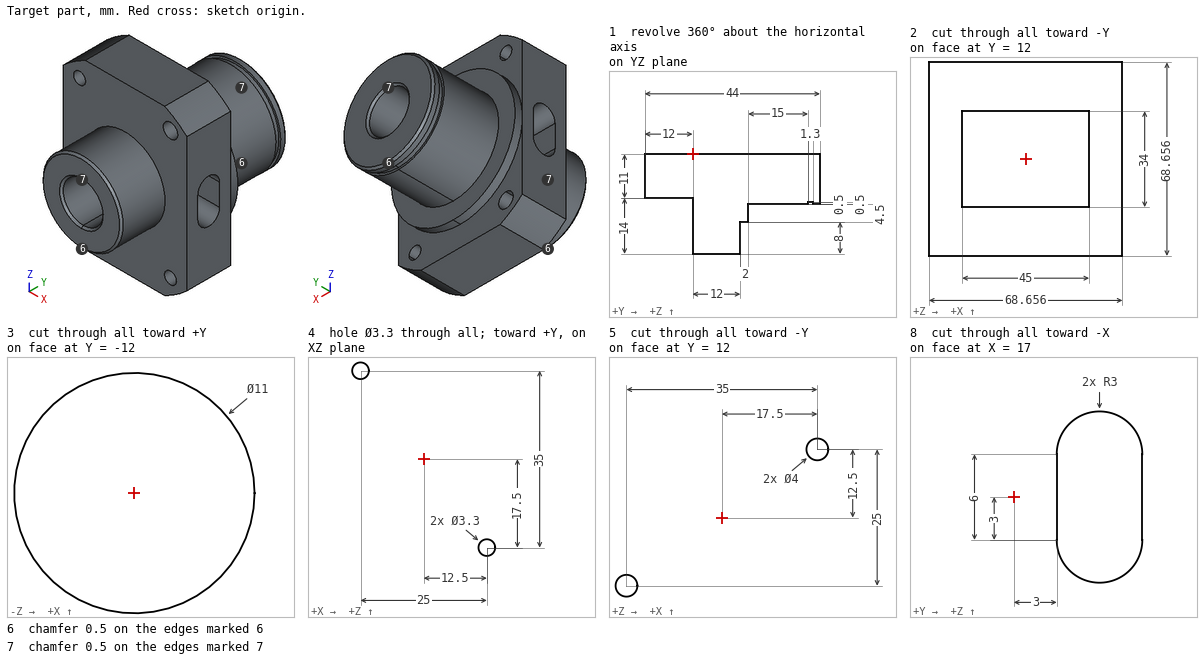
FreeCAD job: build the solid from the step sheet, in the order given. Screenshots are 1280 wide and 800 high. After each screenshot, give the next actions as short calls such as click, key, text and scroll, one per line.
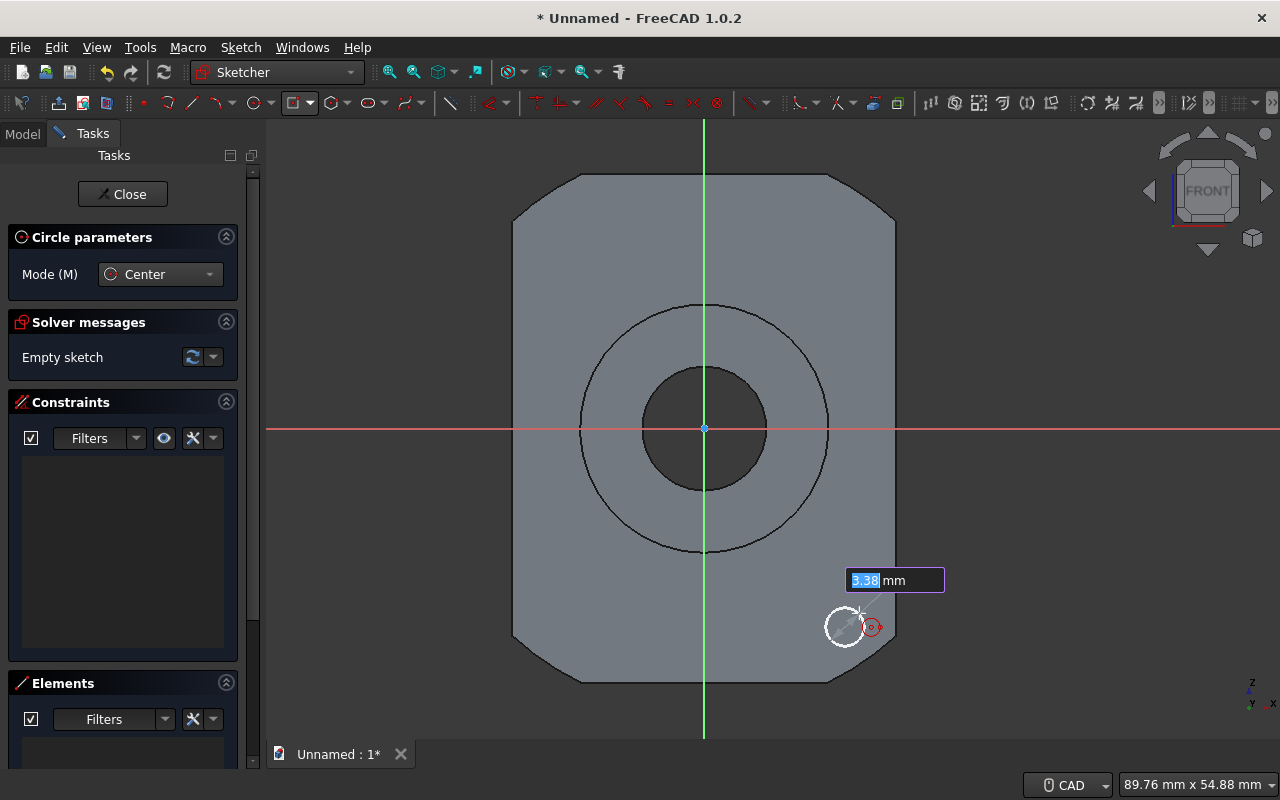
text(3.3)
key(Return)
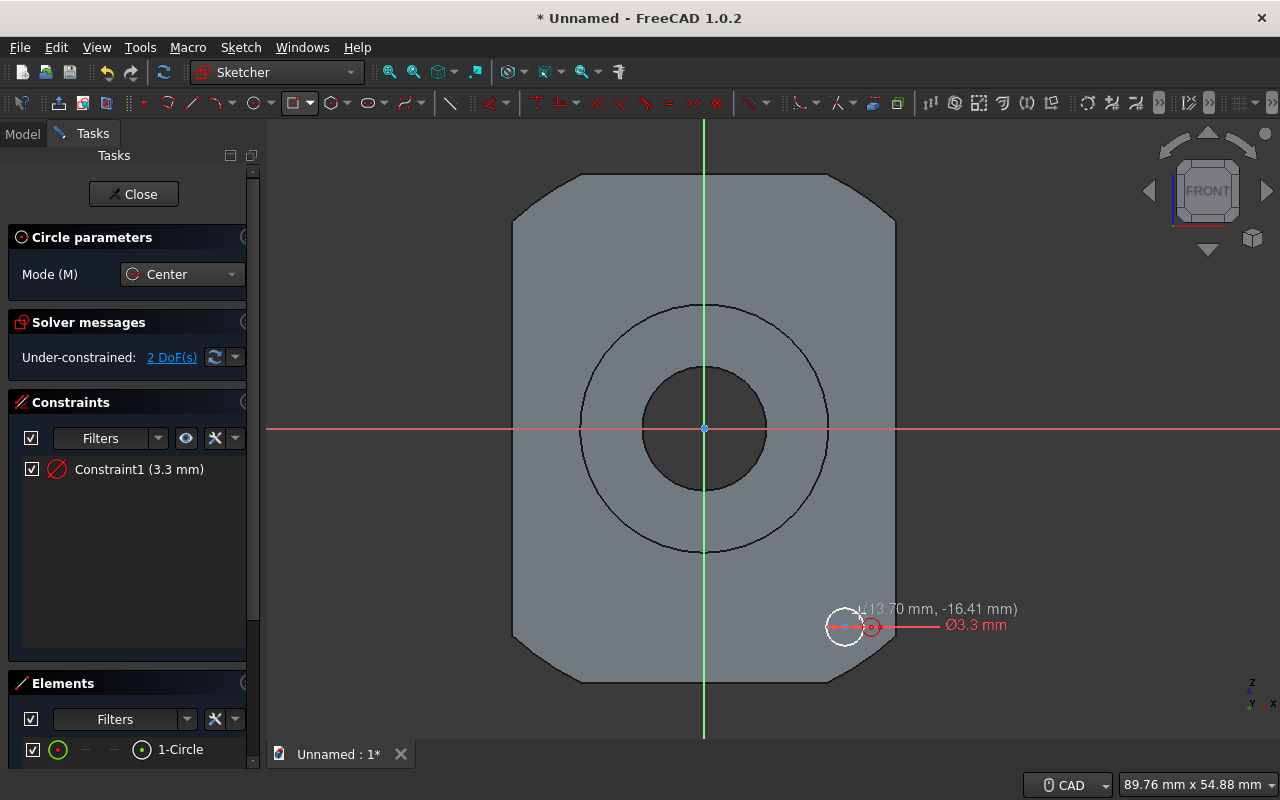
click(563, 231)
move(576, 218)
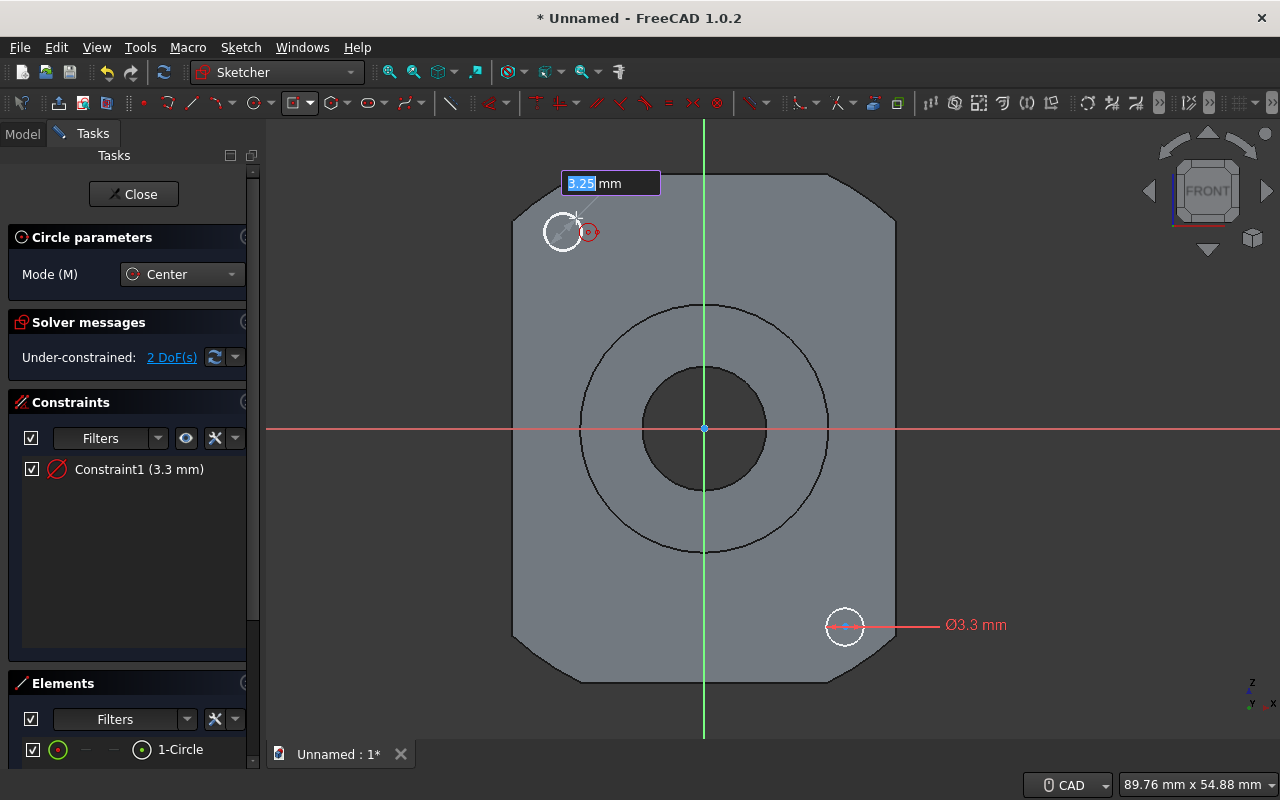
text(3.3)
key(Return)
key(Escape)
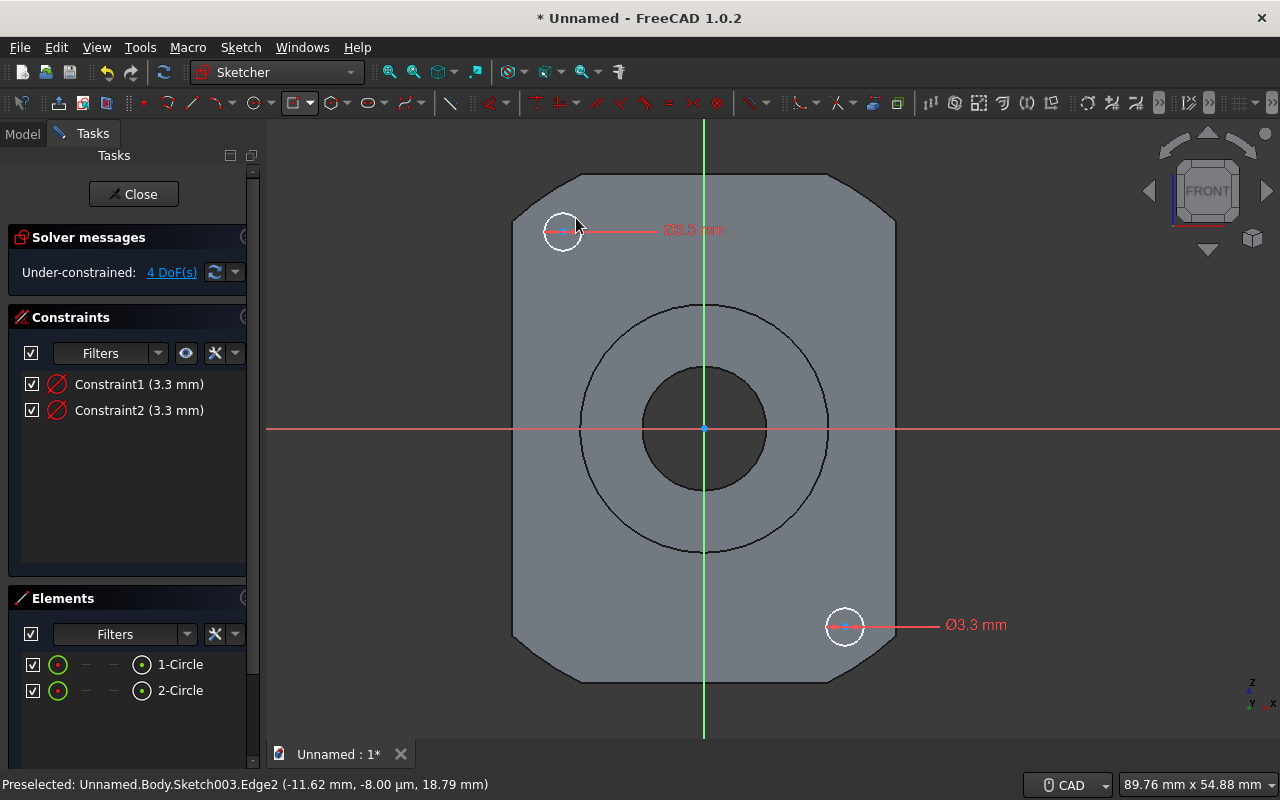
click(490, 104)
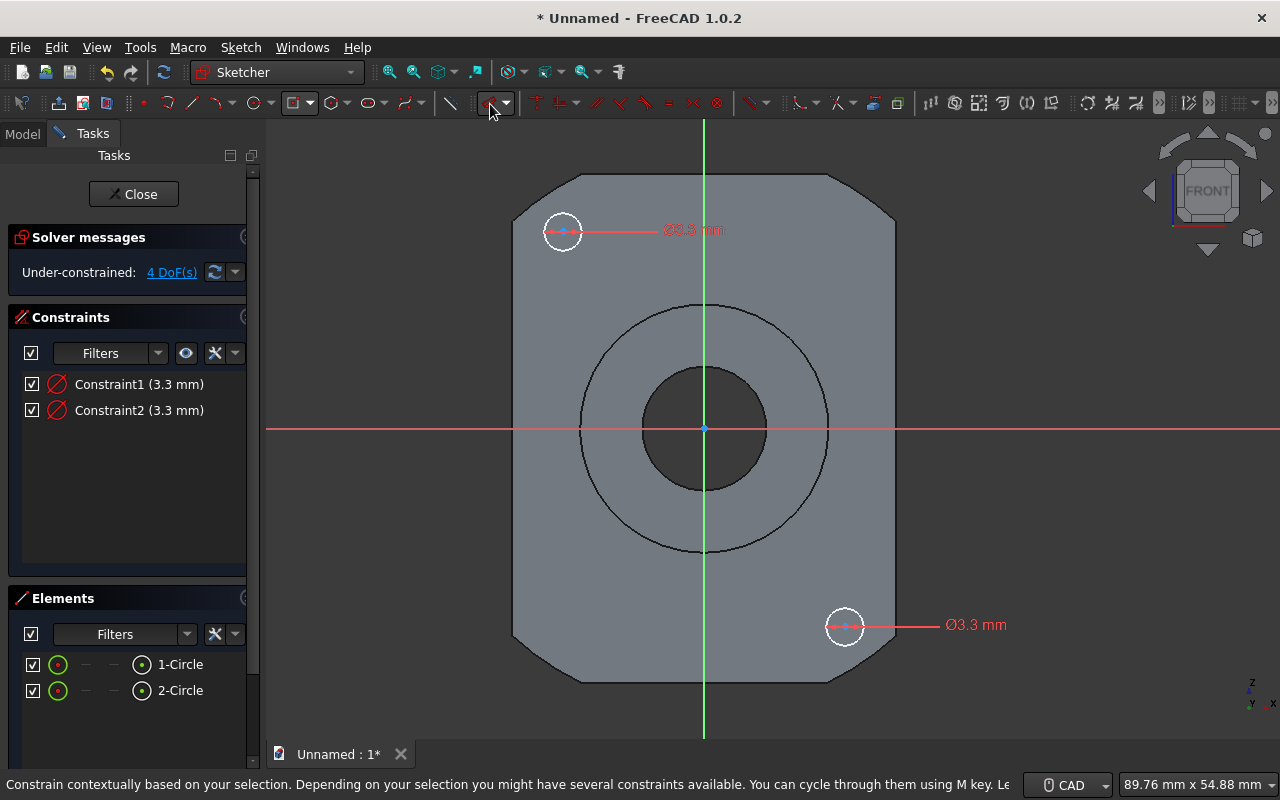
click(845, 627)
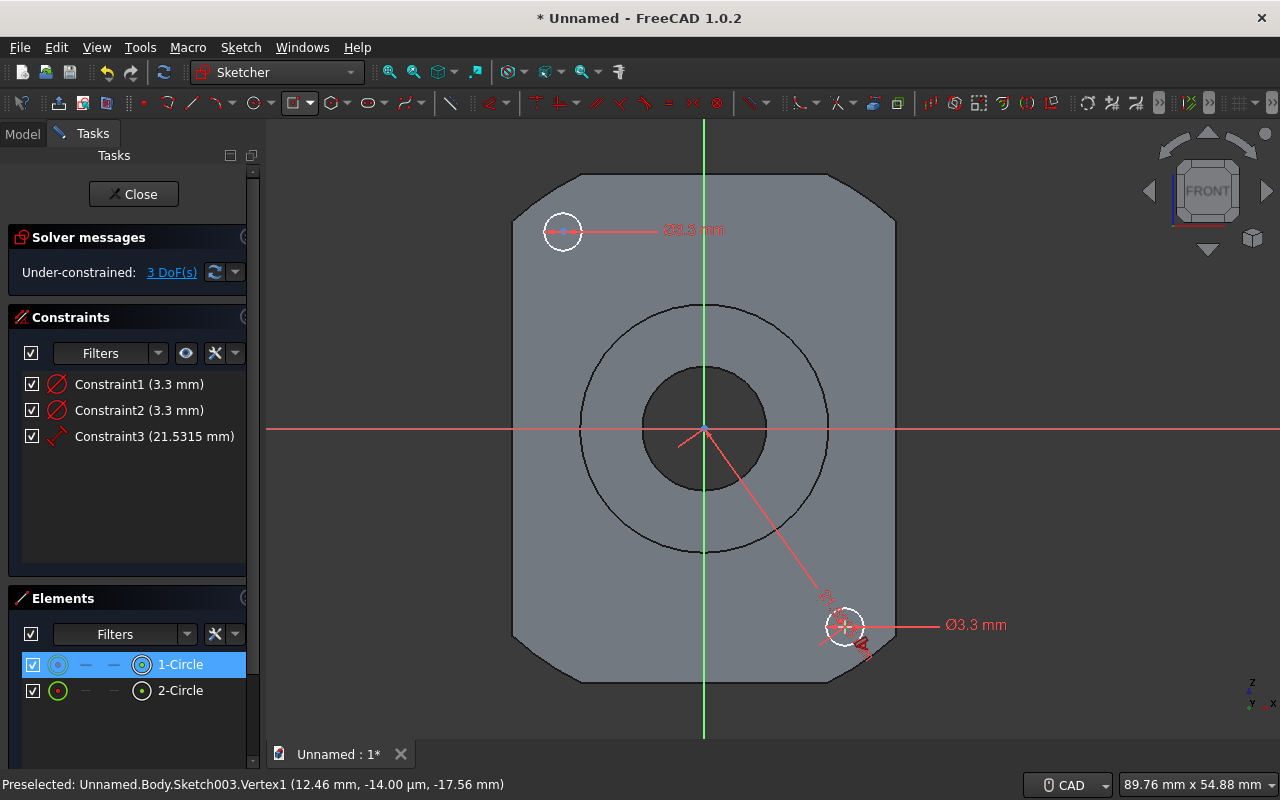
click(563, 232)
click(639, 661)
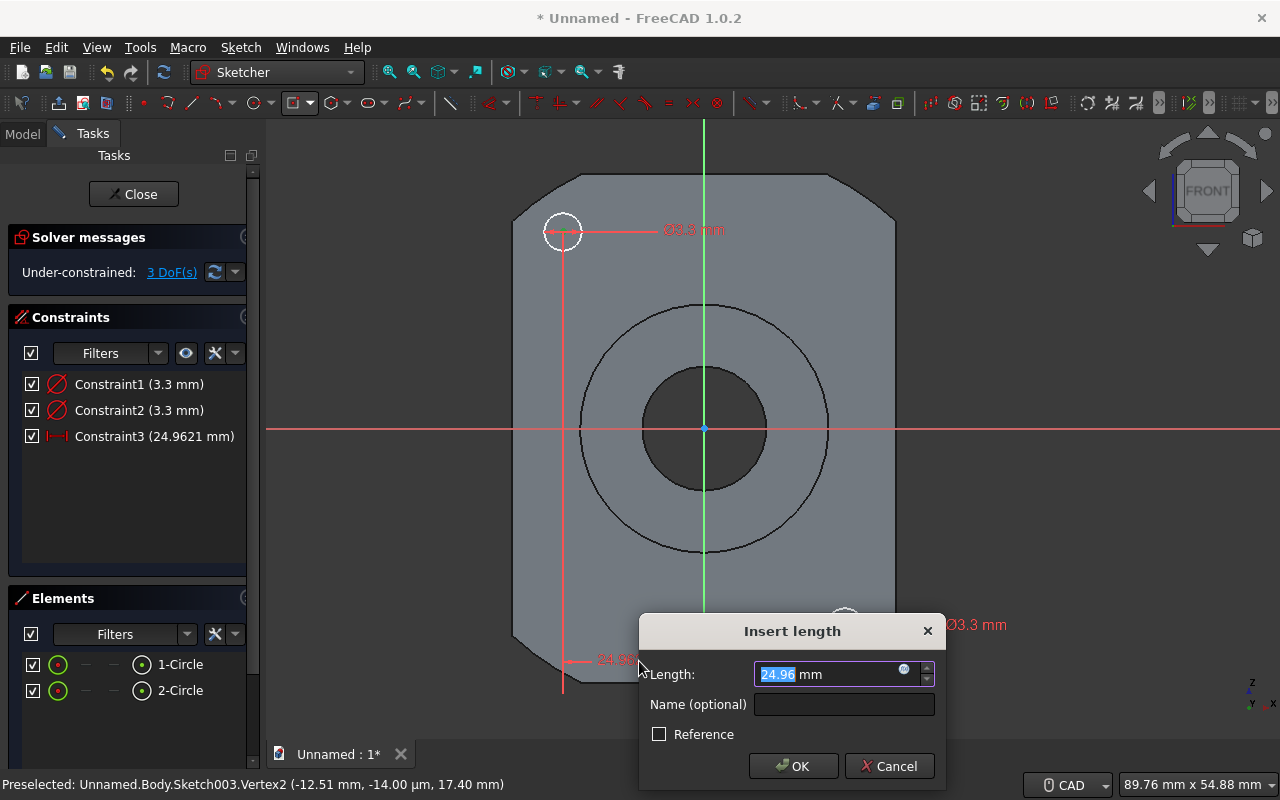
text(25)
key(Return)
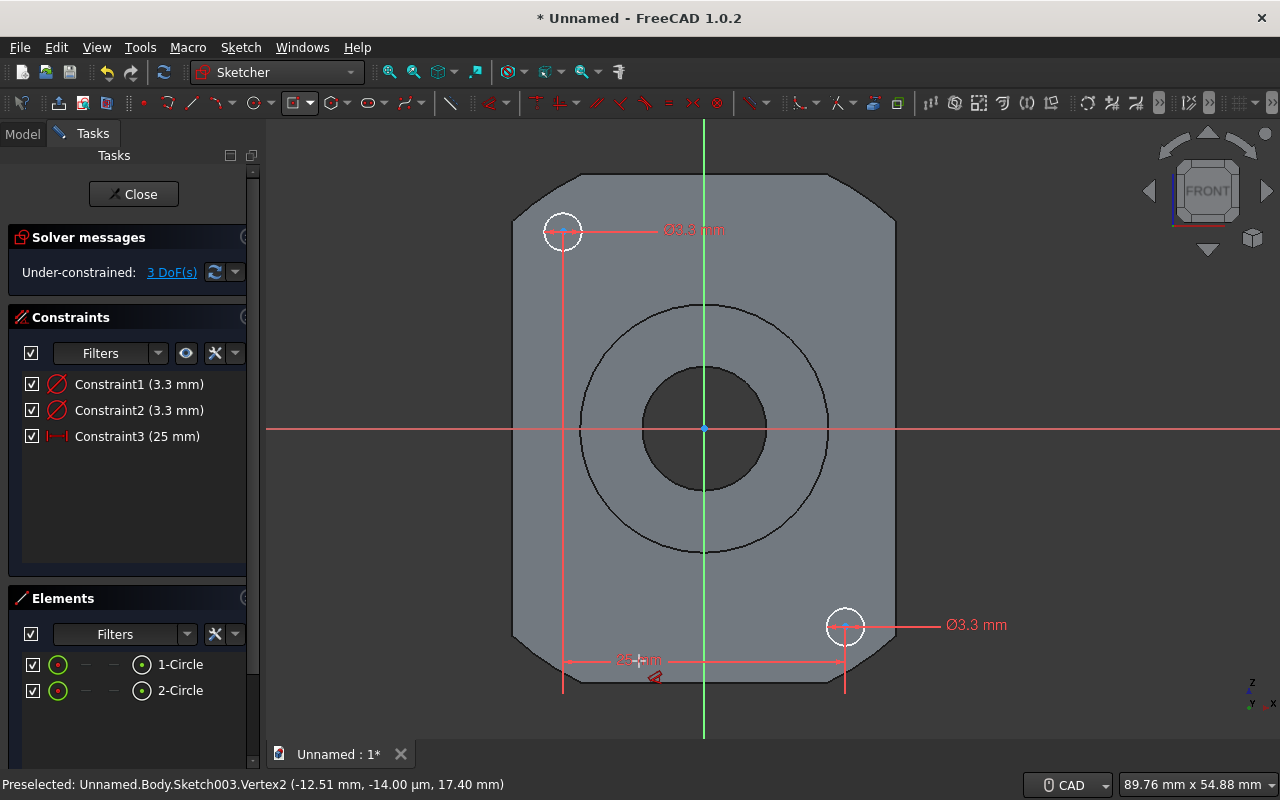
click(845, 627)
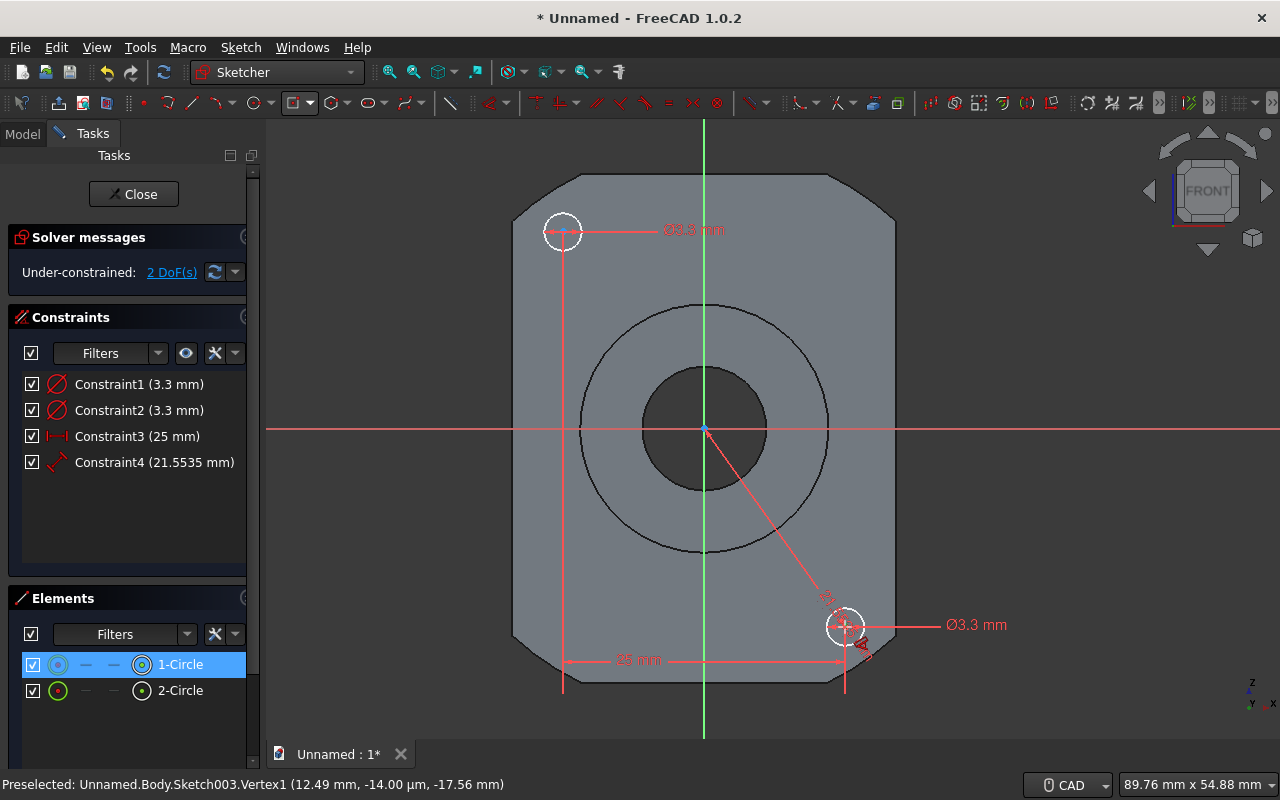
click(563, 232)
click(529, 339)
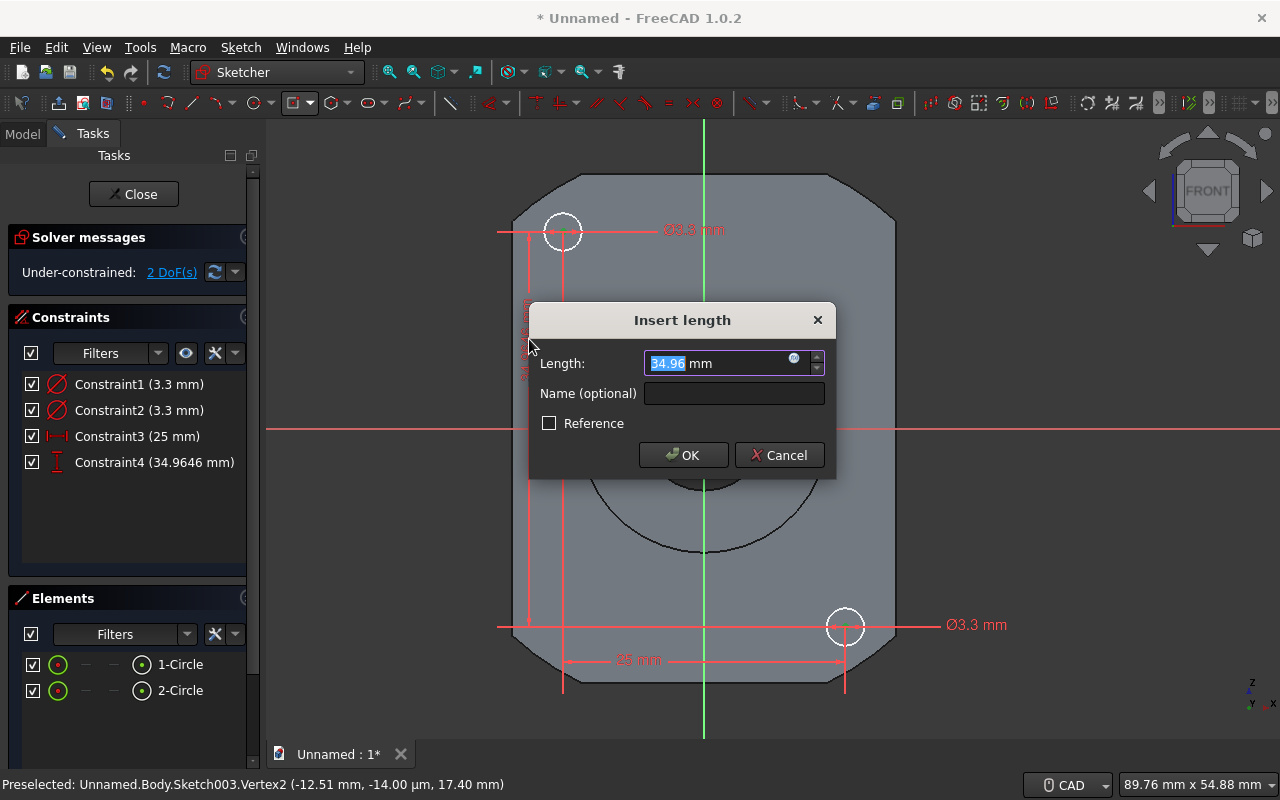
text(35)
key(Return)